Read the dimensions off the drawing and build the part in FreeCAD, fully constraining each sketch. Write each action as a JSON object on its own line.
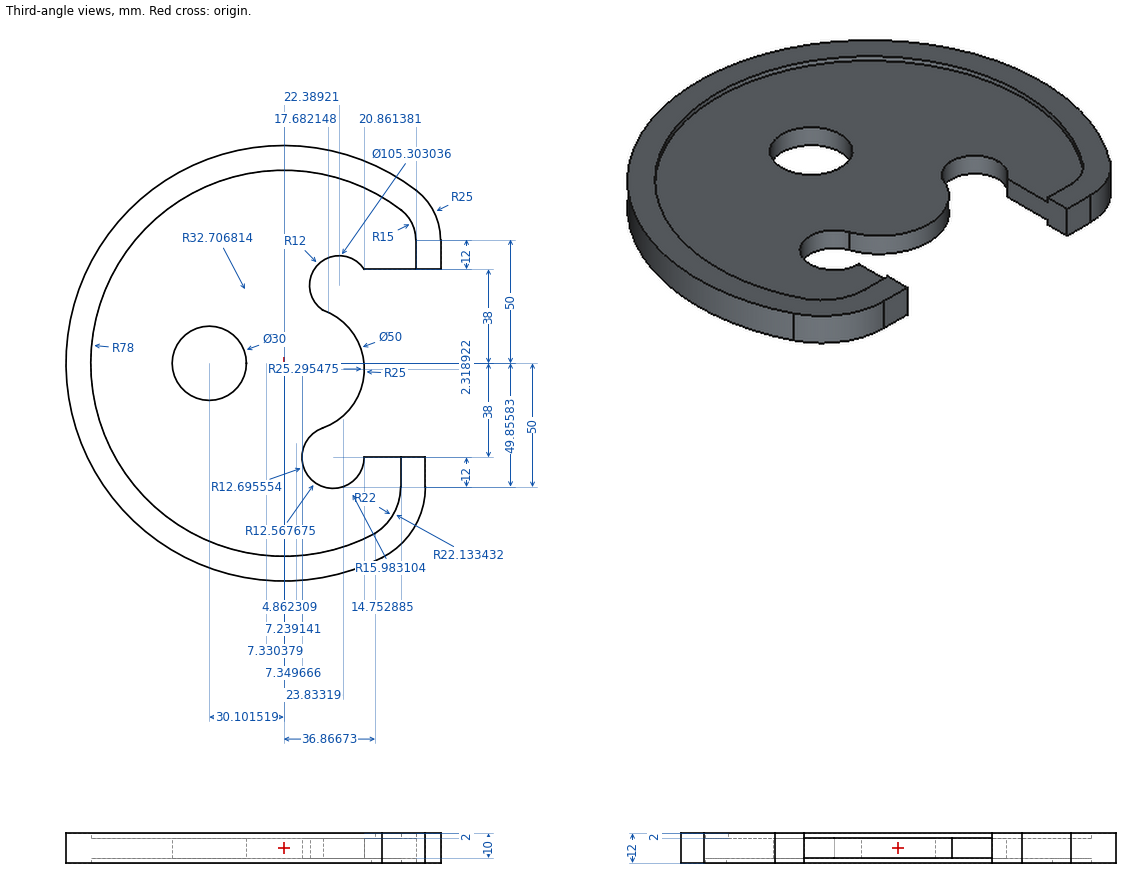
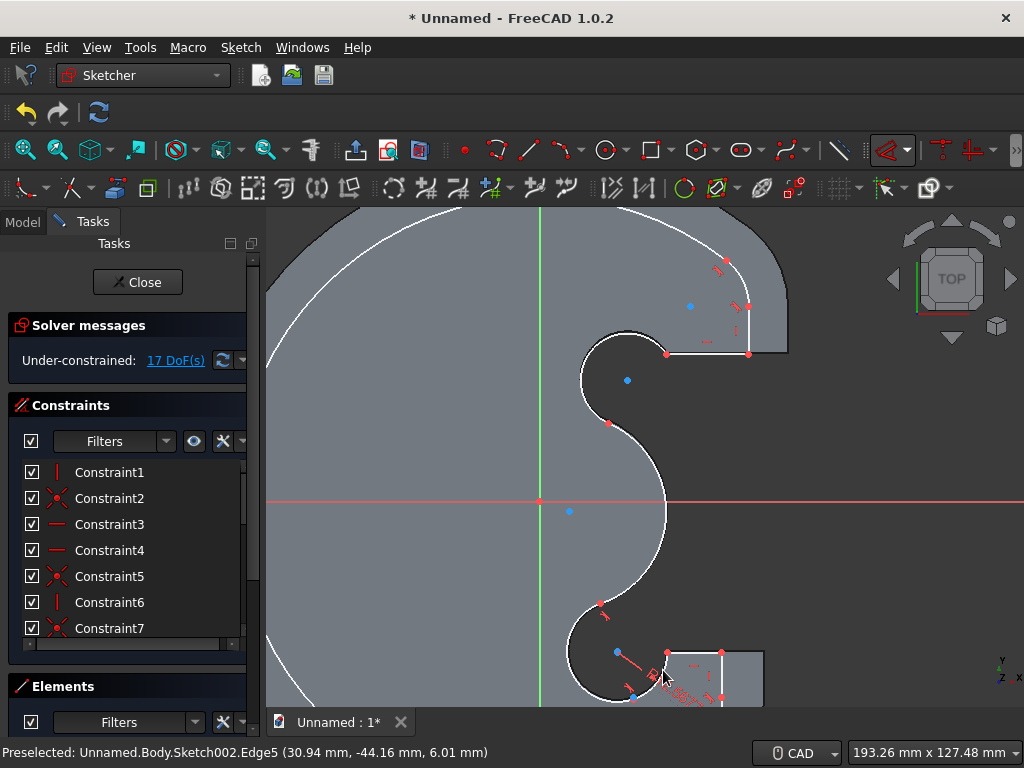
{"action": "left_click", "coordinate": [569, 637]}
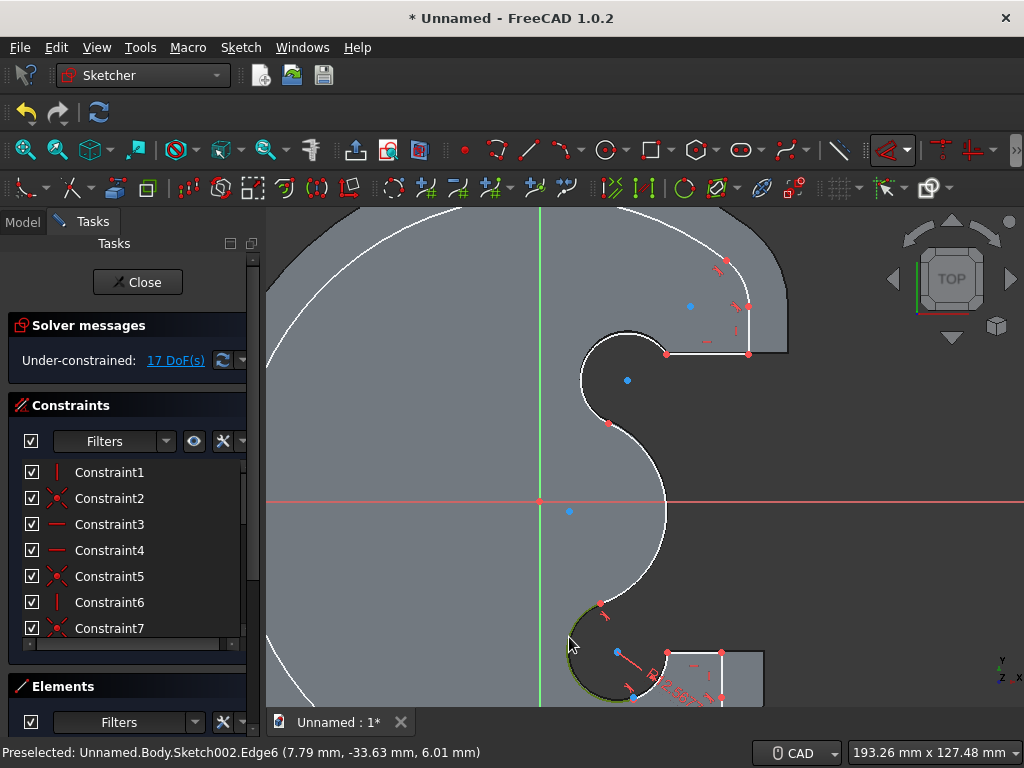
{"action": "key", "text": "k r"}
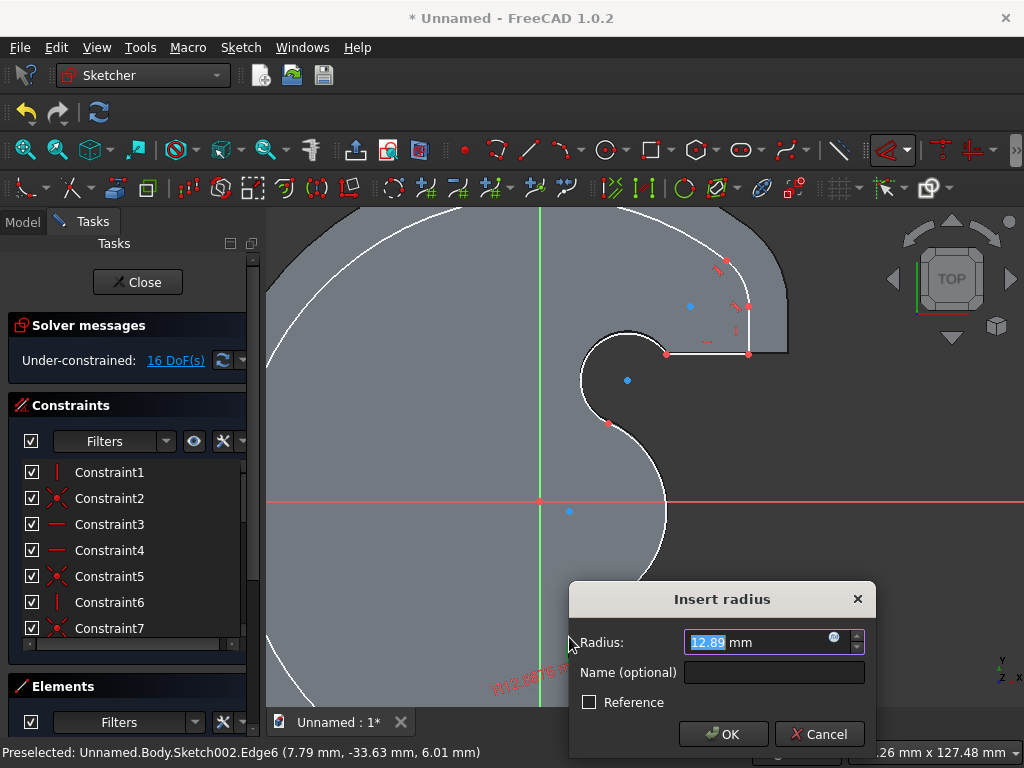
{"action": "type", "text": "12.695554"}
{"action": "key", "text": "Return"}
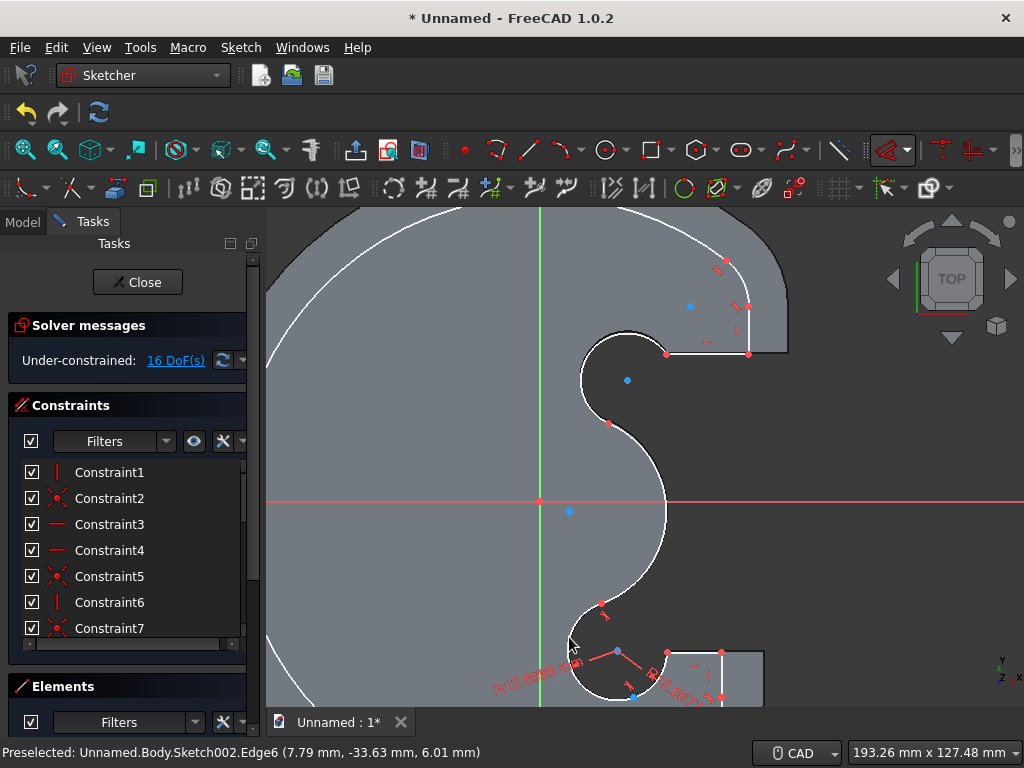
{"action": "left_click", "coordinate": [653, 560]}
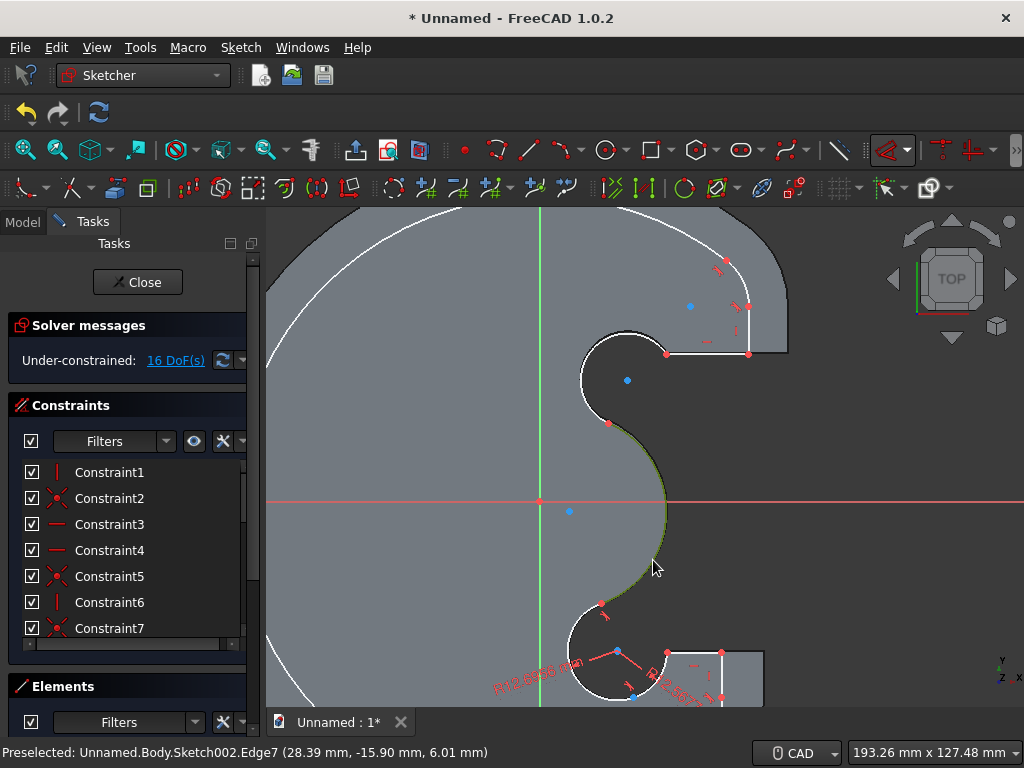
{"action": "left_click", "coordinate": [910, 150]}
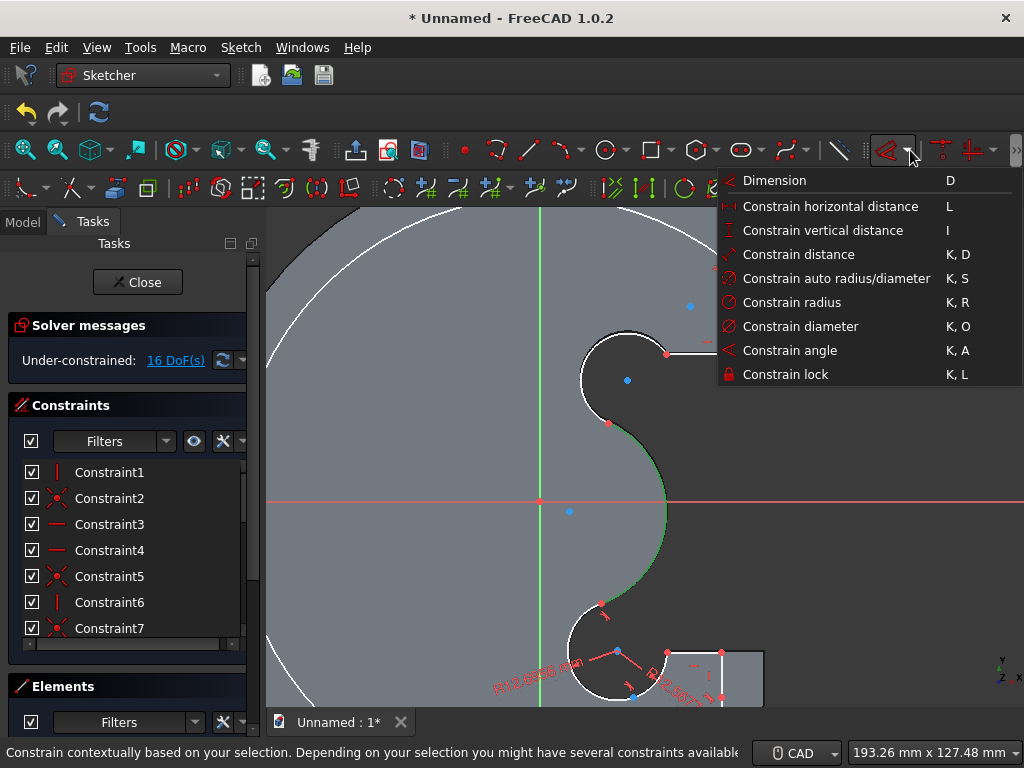
{"action": "left_click", "coordinate": [870, 302]}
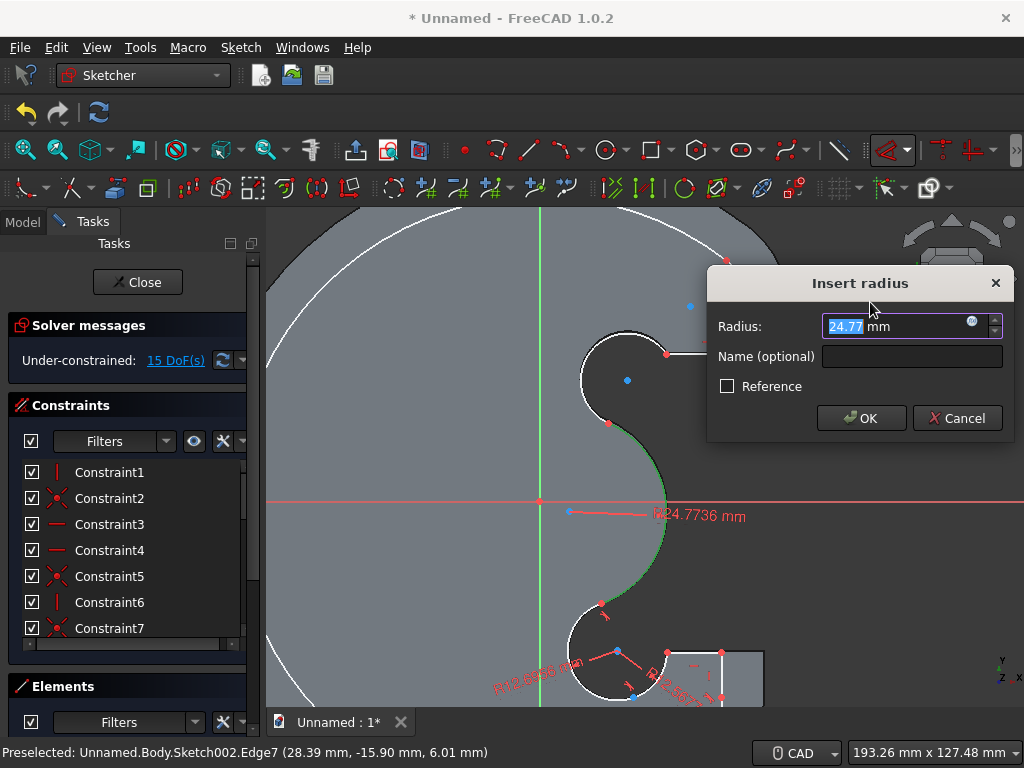
{"action": "type", "text": "25"}
{"action": "key", "text": "Return"}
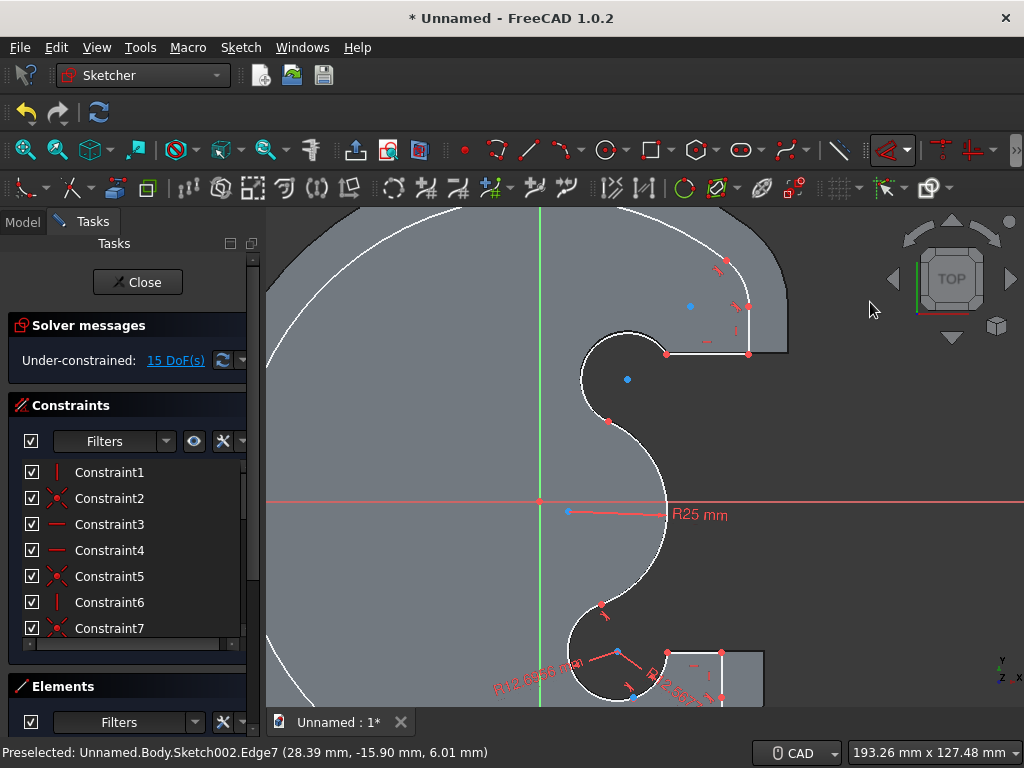
{"action": "left_click", "coordinate": [622, 334]}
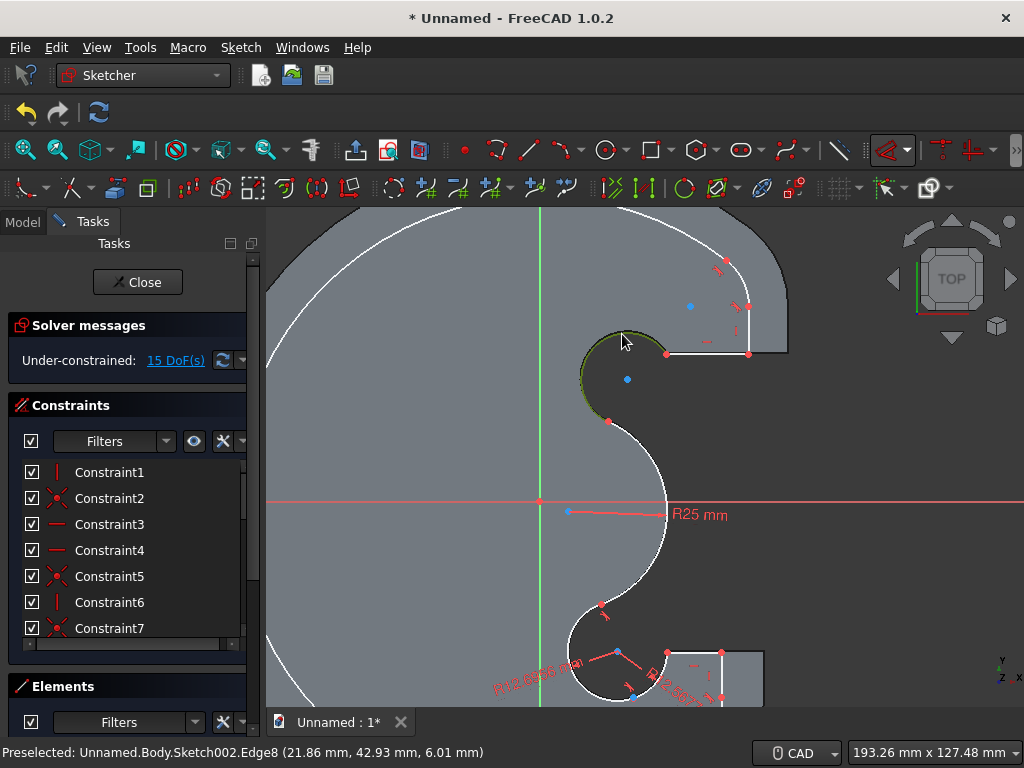
{"action": "key", "text": "k r"}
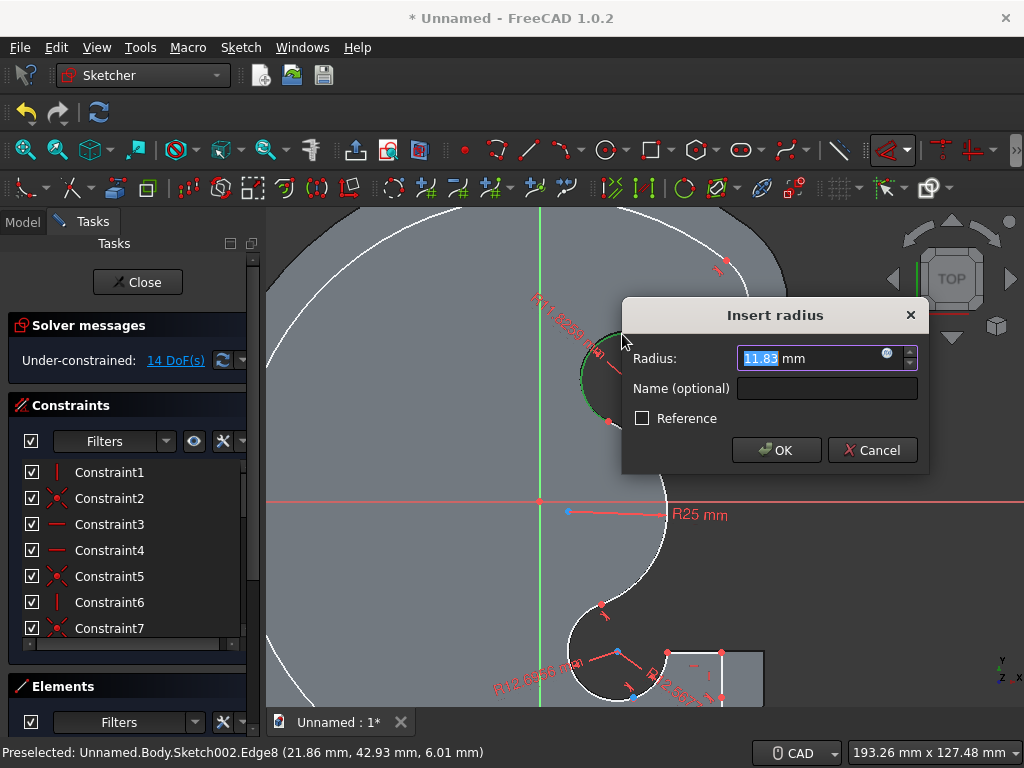
{"action": "type", "text": "12"}
{"action": "key", "text": "Return"}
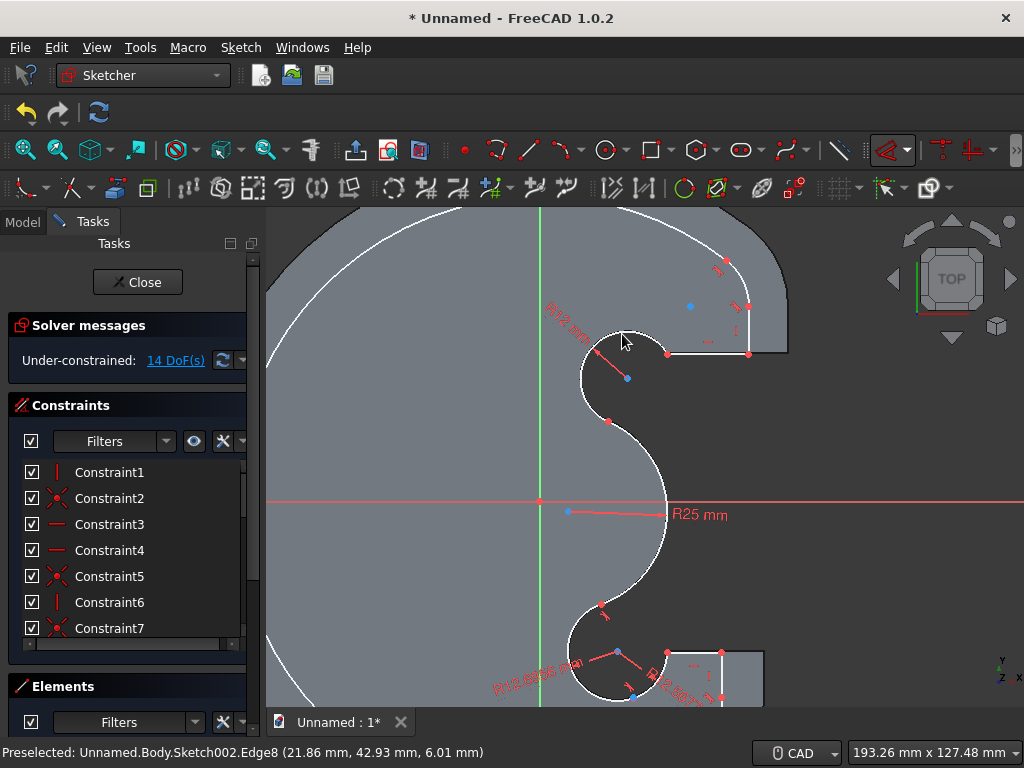
{"action": "left_click", "coordinate": [747, 291]}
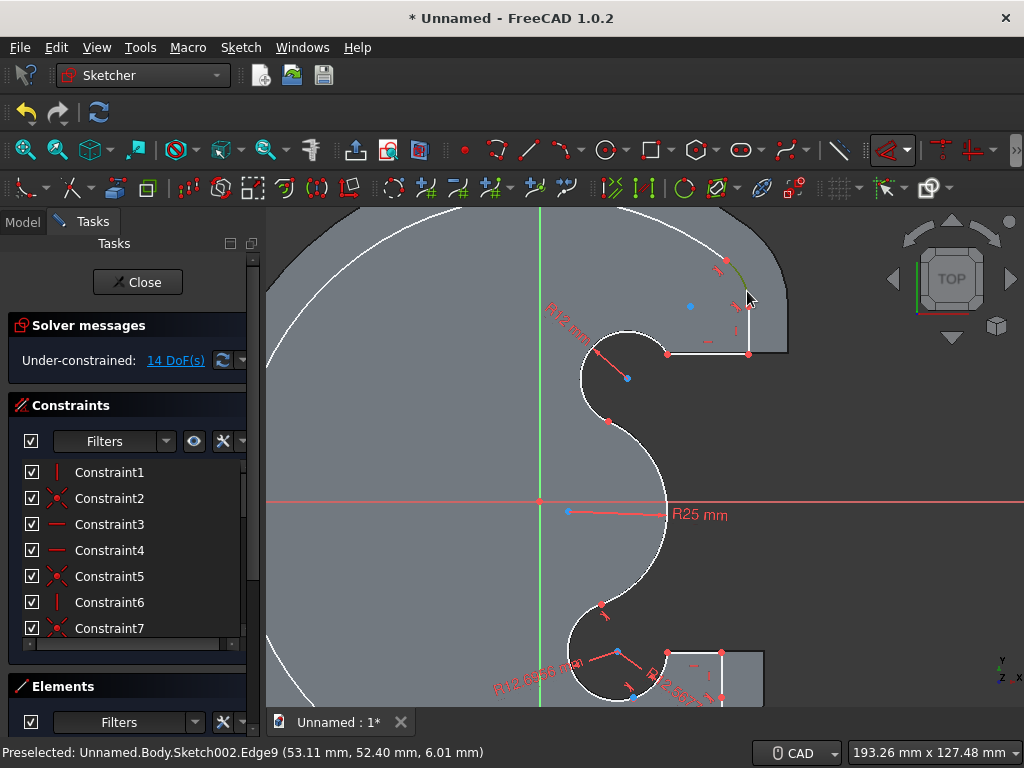
{"action": "key", "text": "k r"}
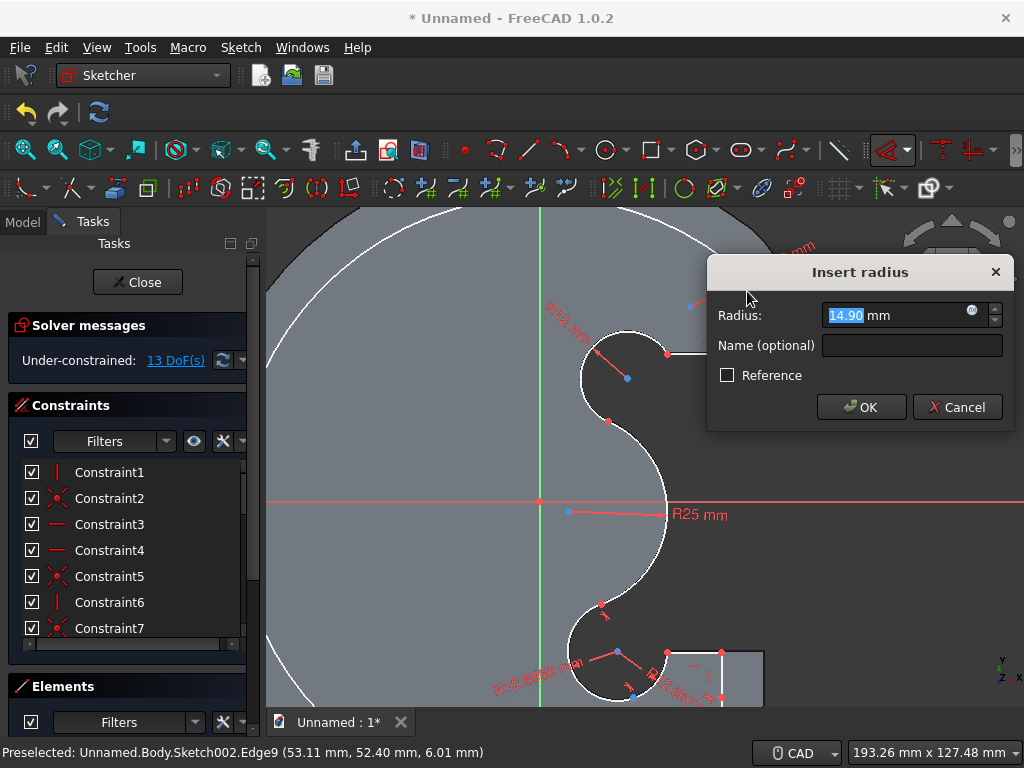
{"action": "type", "text": "15"}
{"action": "key", "text": "Return"}